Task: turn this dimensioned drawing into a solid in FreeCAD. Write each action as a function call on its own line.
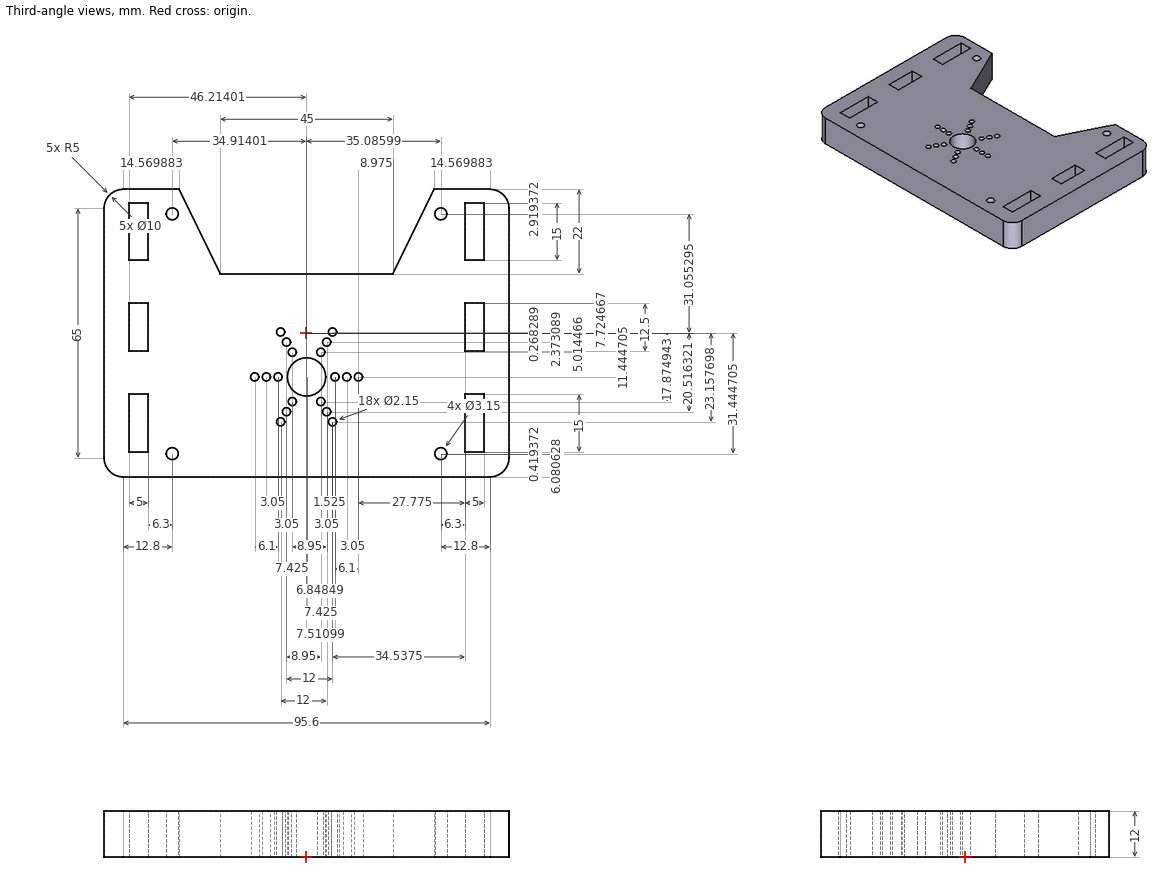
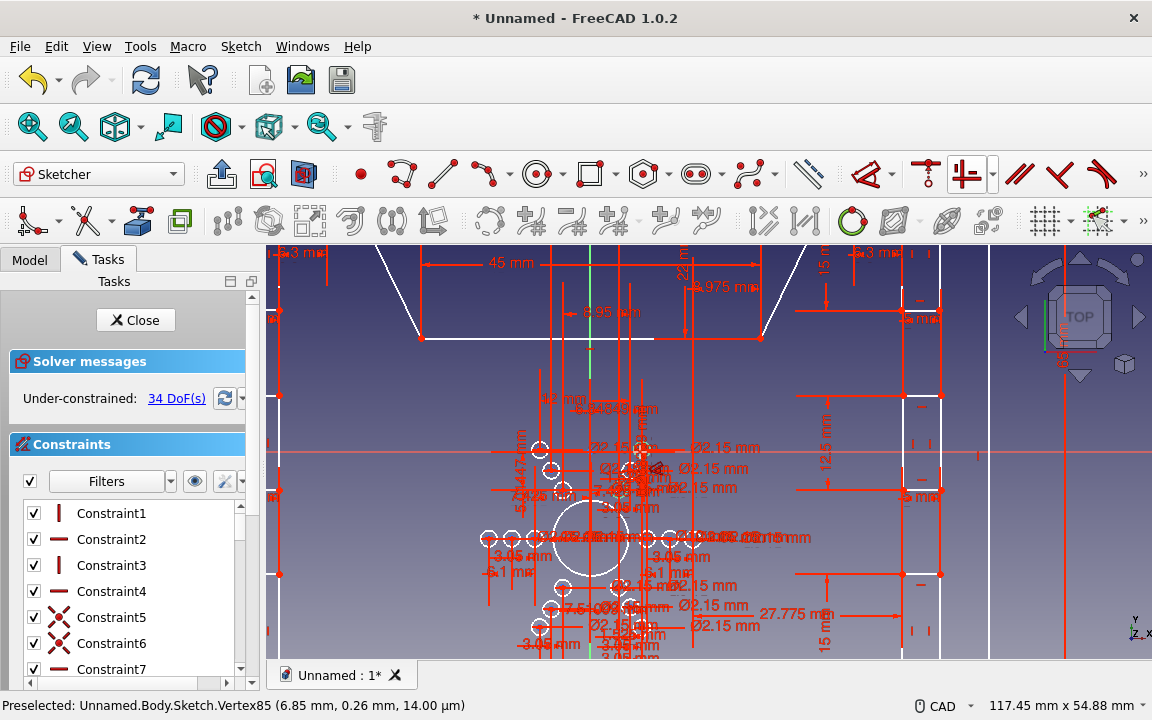
scroll(681, 452, down, 4)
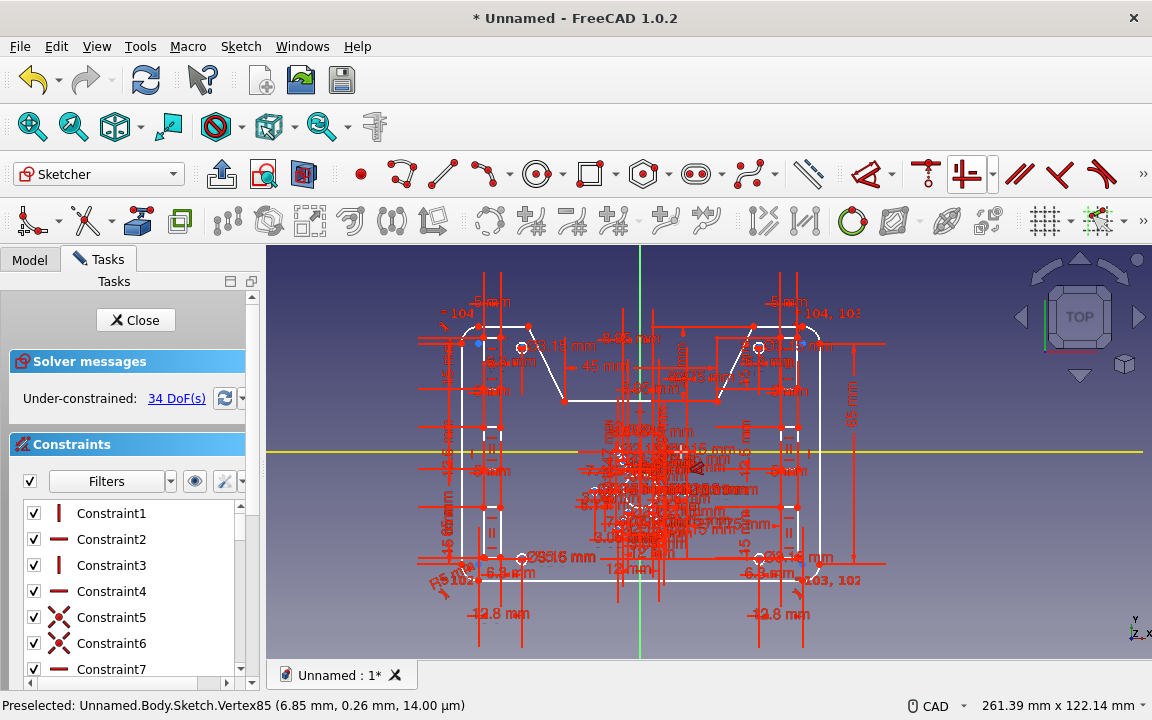
scroll(659, 461, up, 8)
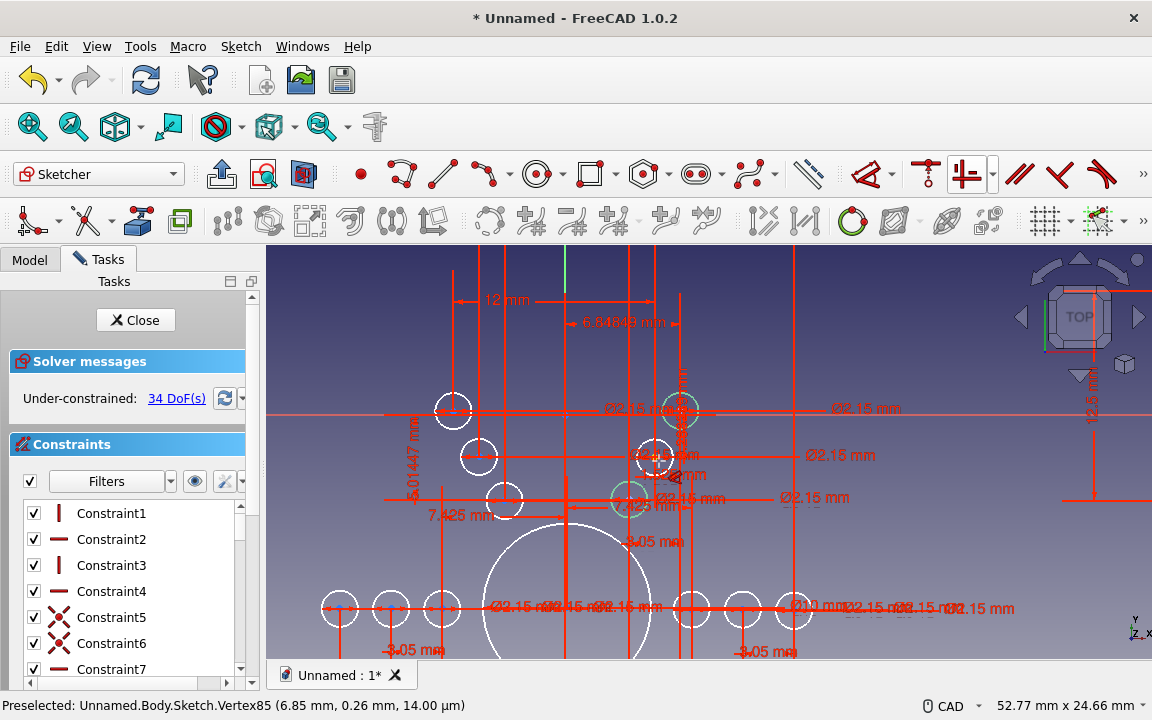
click(655, 457)
click(689, 446)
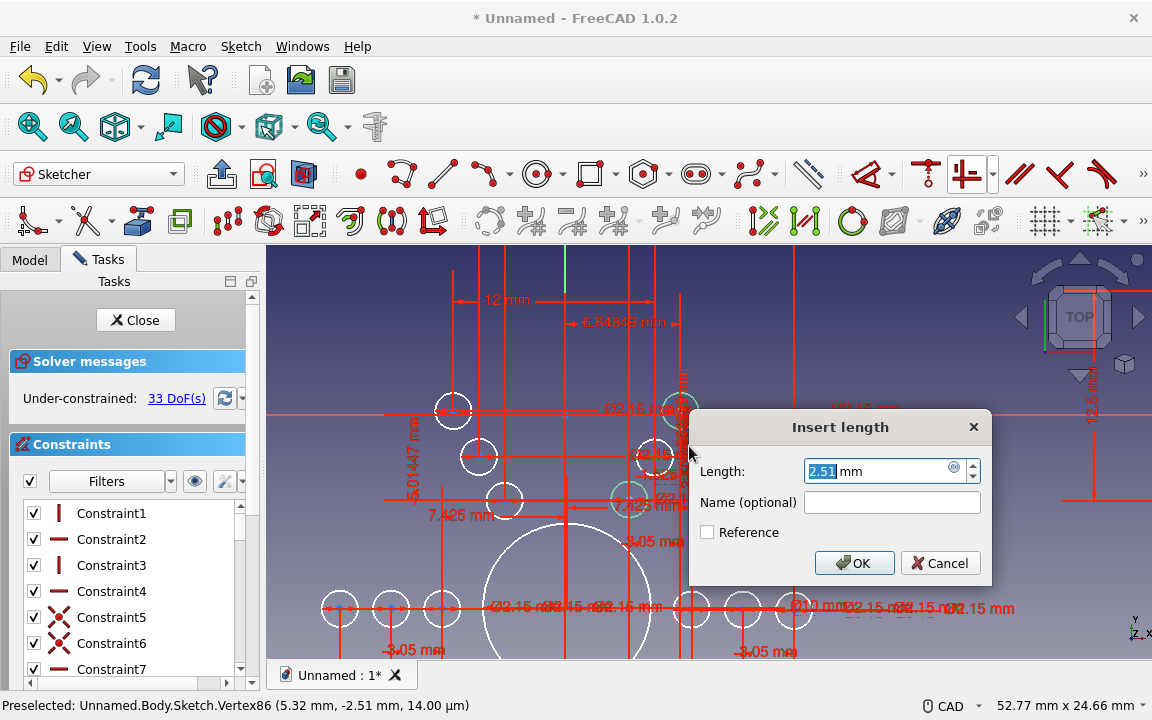
text(2.373089)
key(Return)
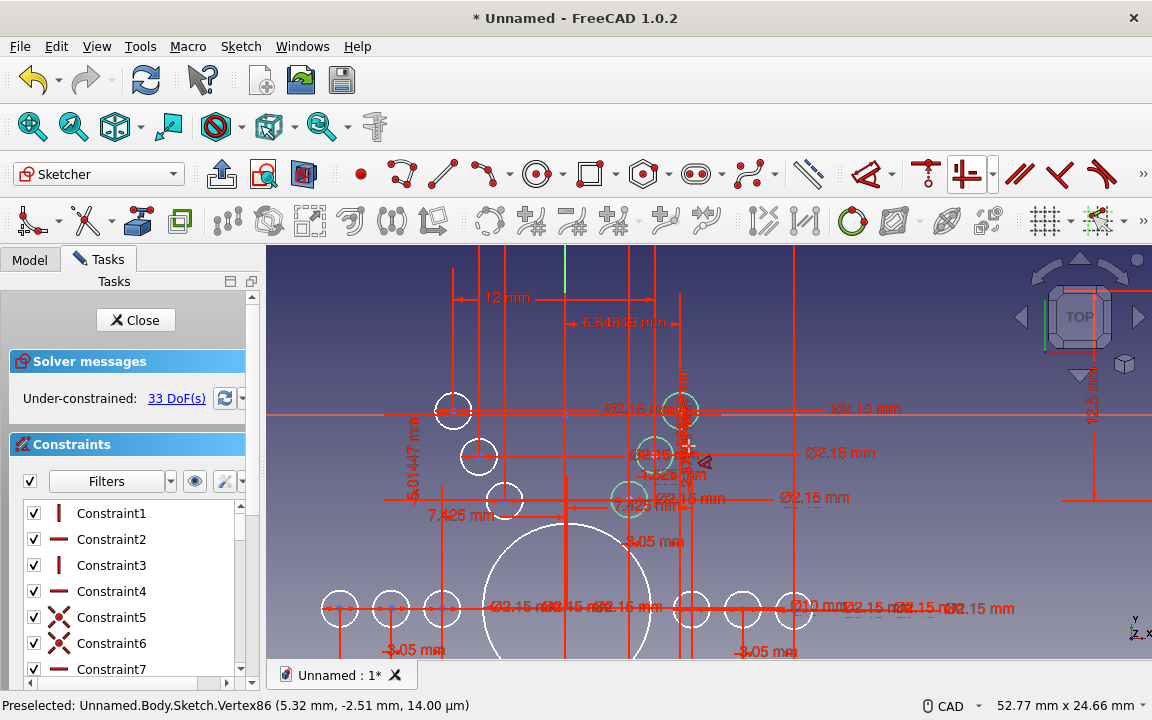
click(505, 501)
click(471, 488)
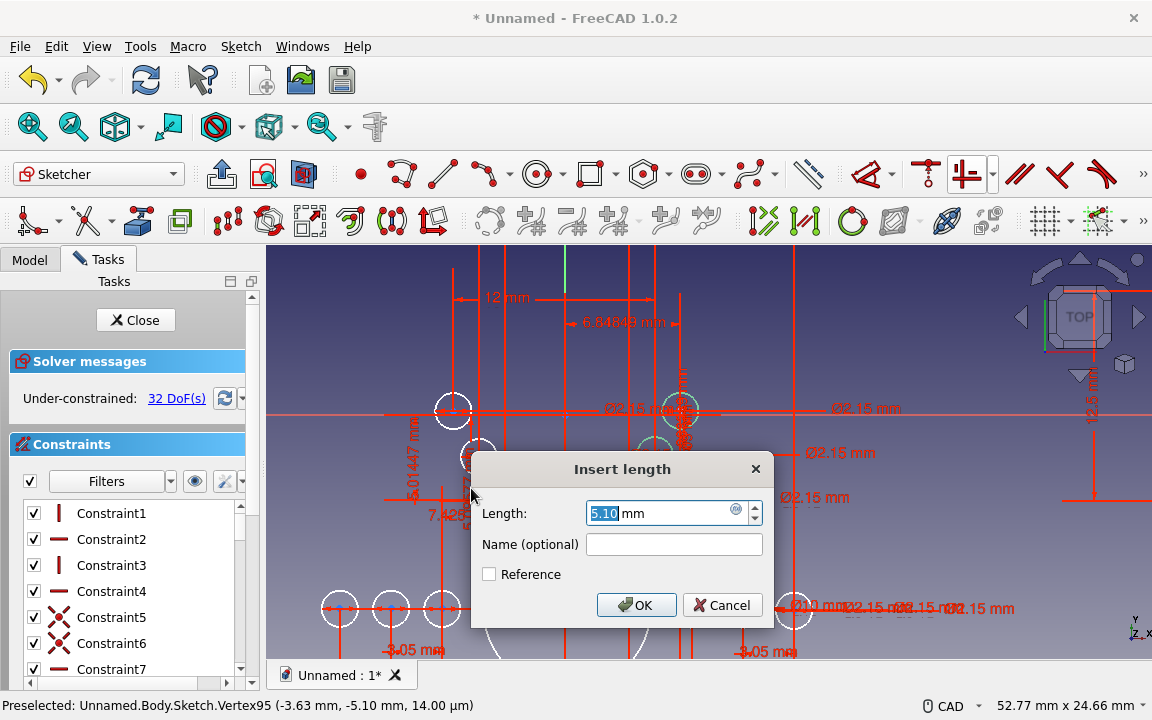
text(5.014466)
key(Return)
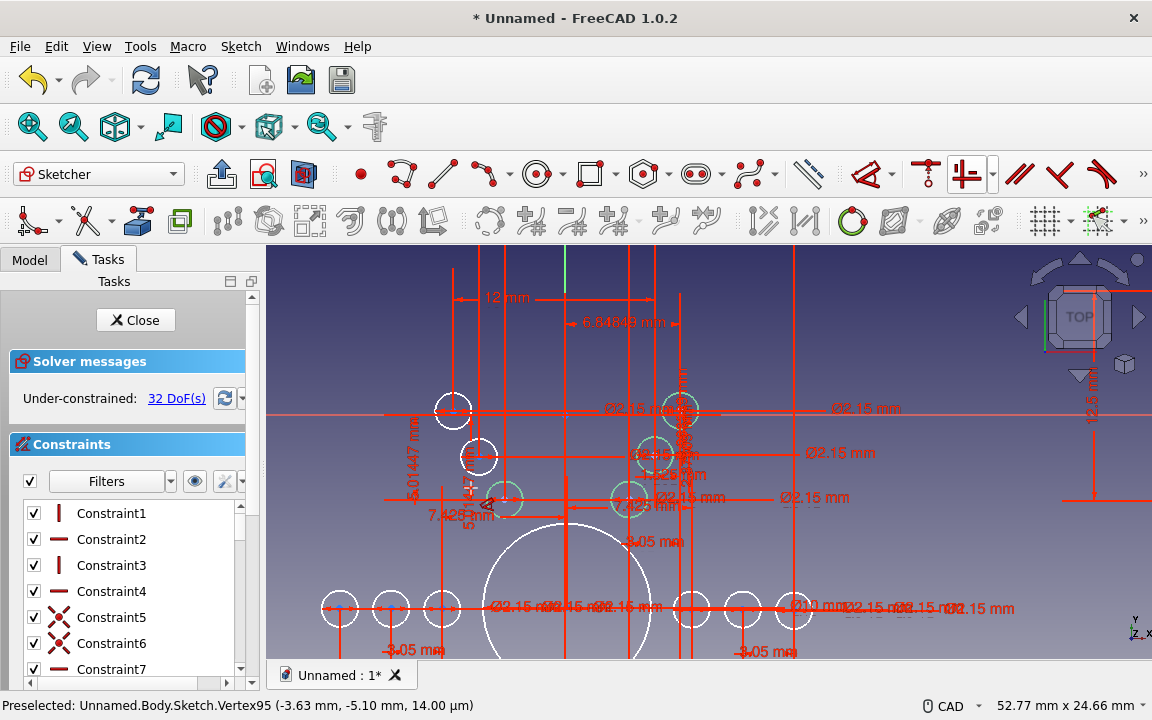
click(479, 457)
click(599, 436)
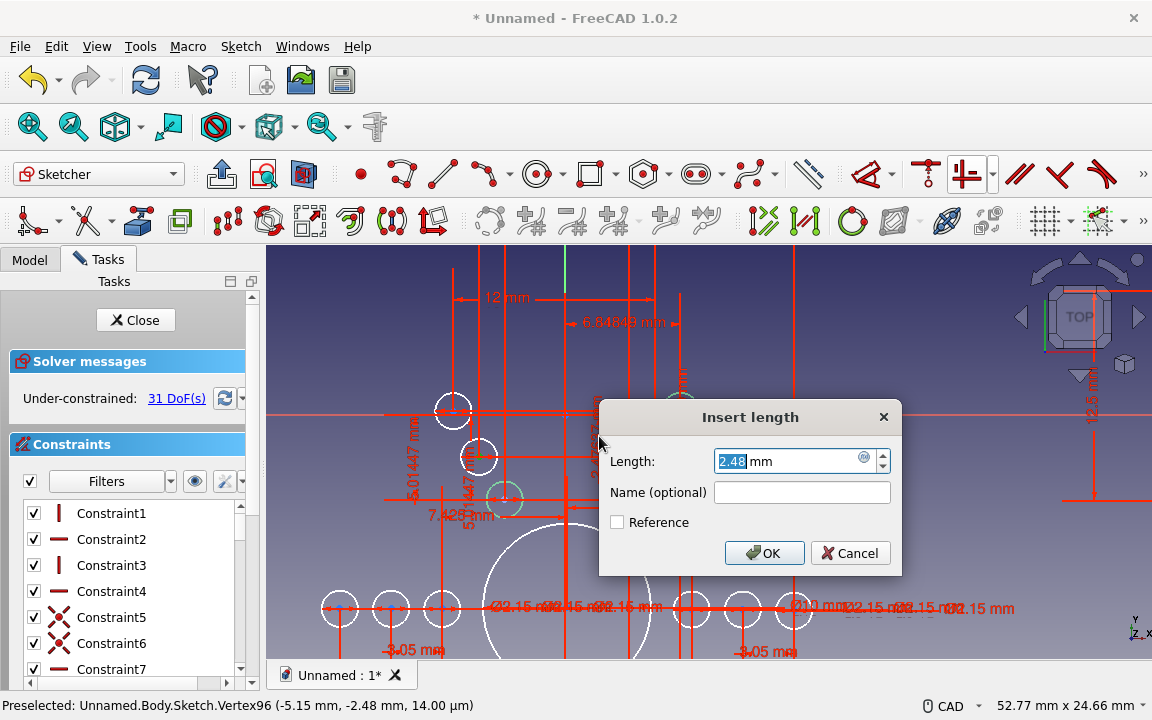
text(2.373089)
key(Return)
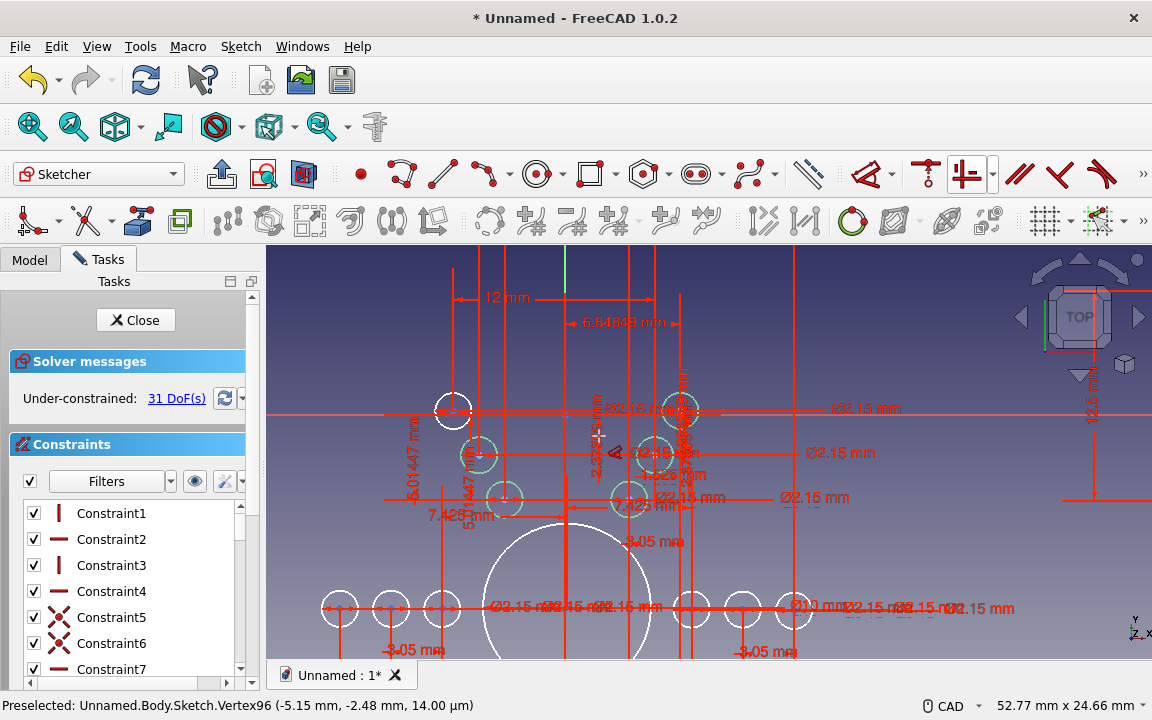
scroll(453, 411, up, 11)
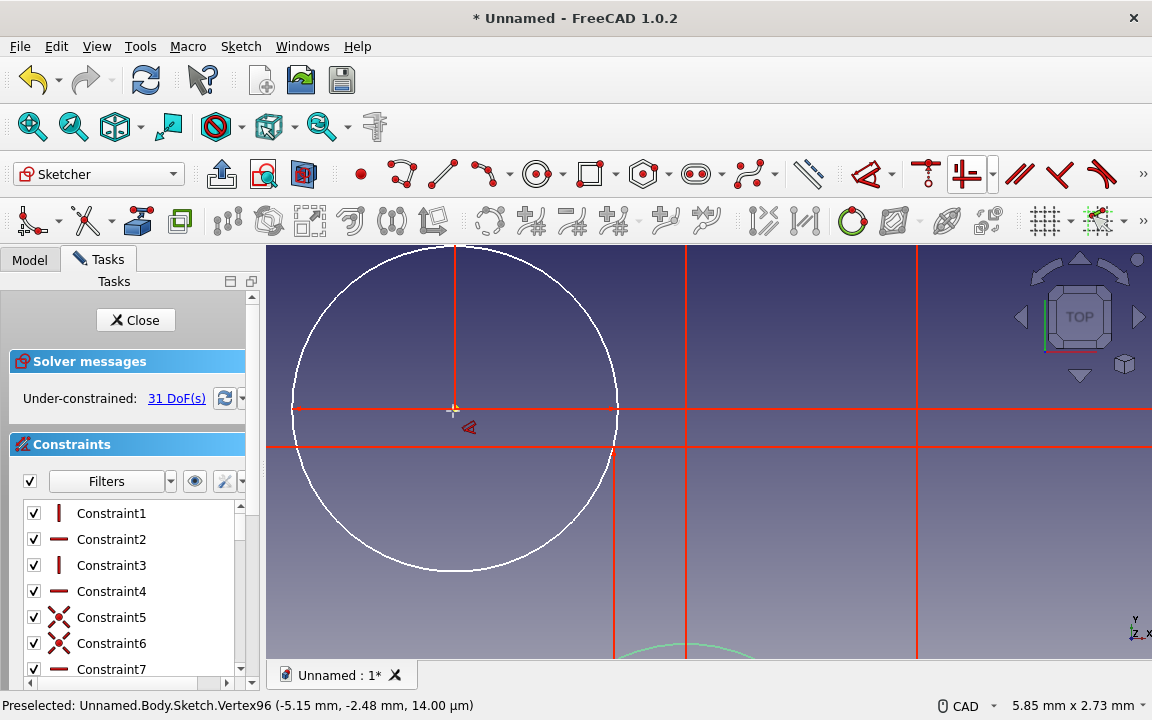
click(455, 409)
click(421, 428)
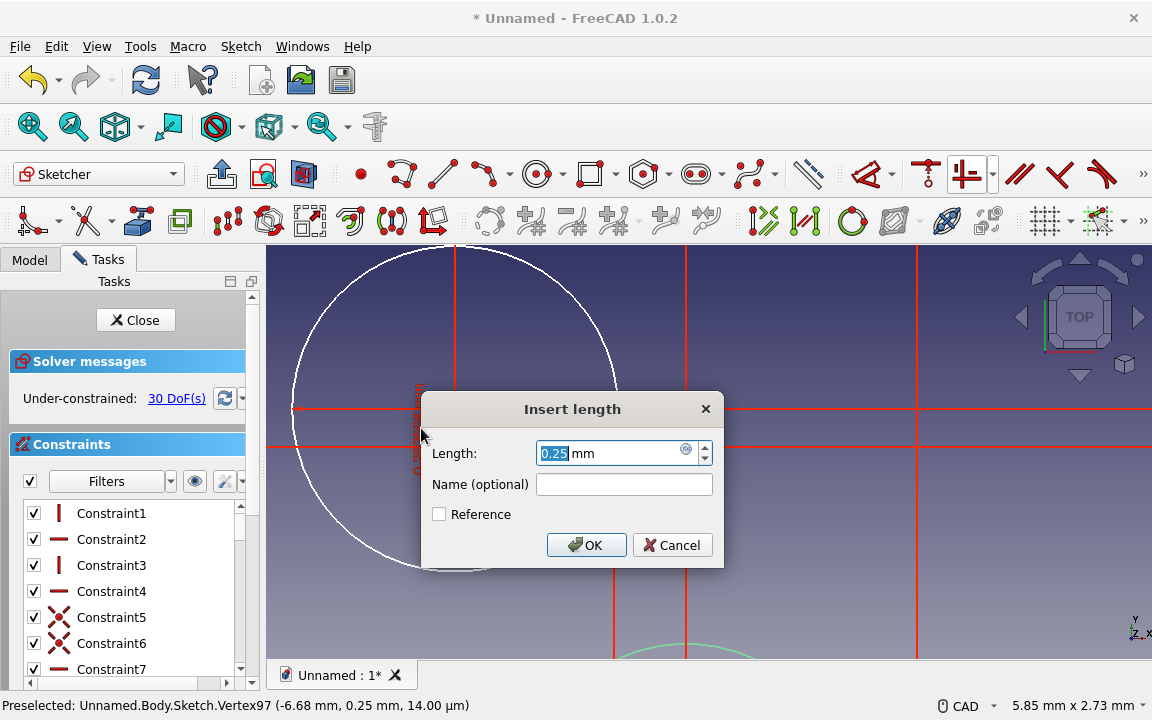
text(0.268289)
key(Return)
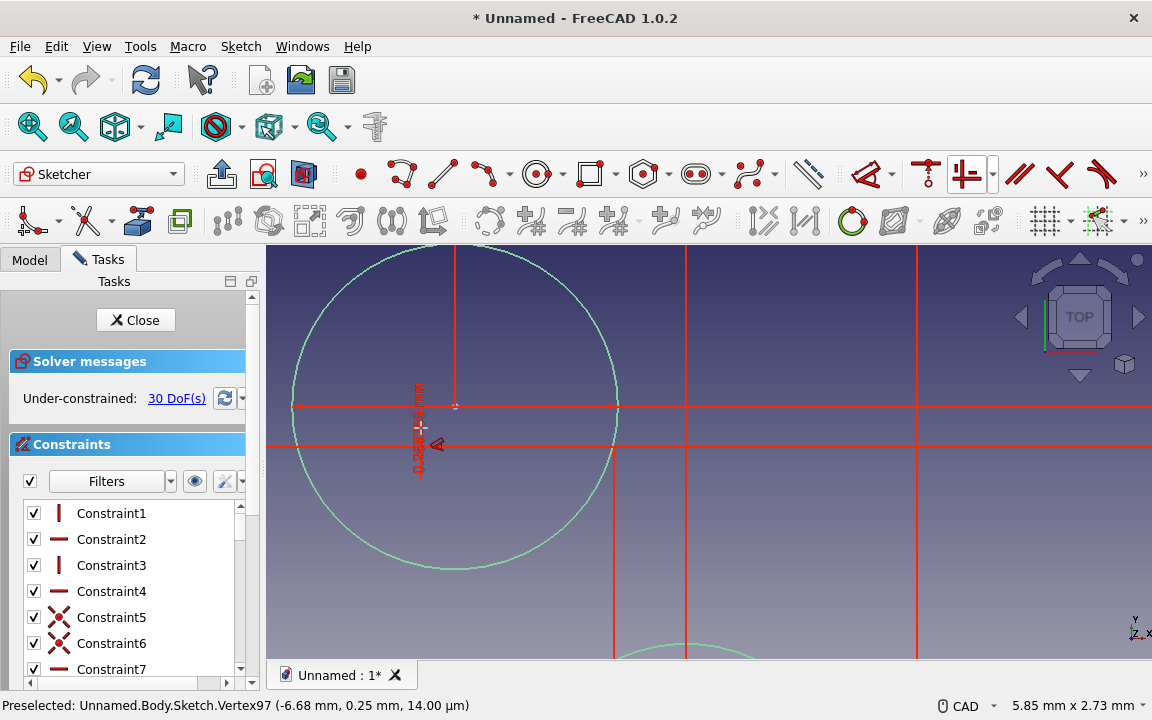
scroll(640, 452, down, 15)